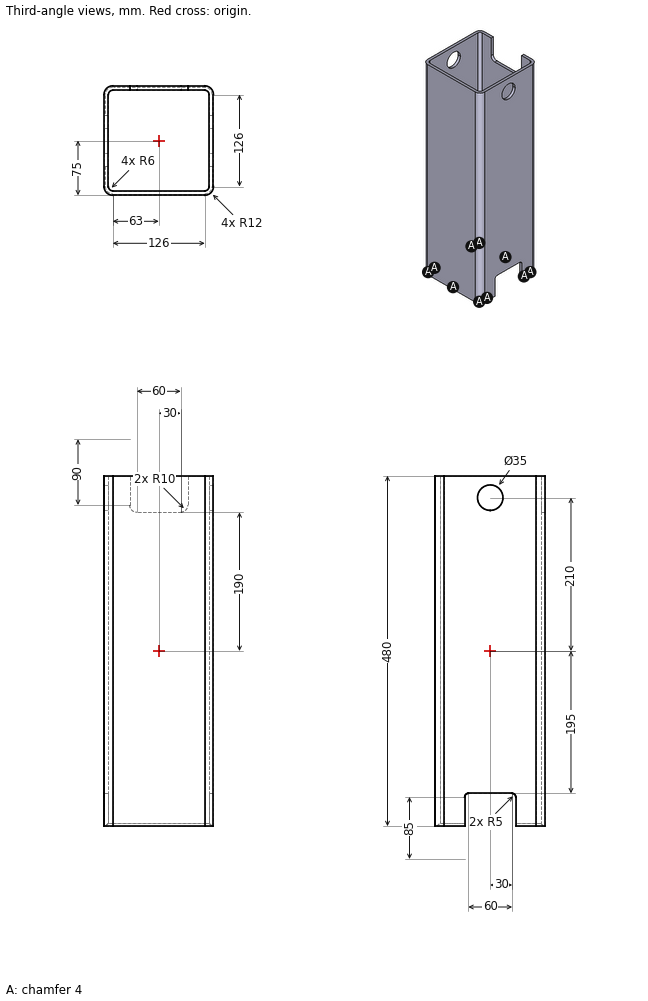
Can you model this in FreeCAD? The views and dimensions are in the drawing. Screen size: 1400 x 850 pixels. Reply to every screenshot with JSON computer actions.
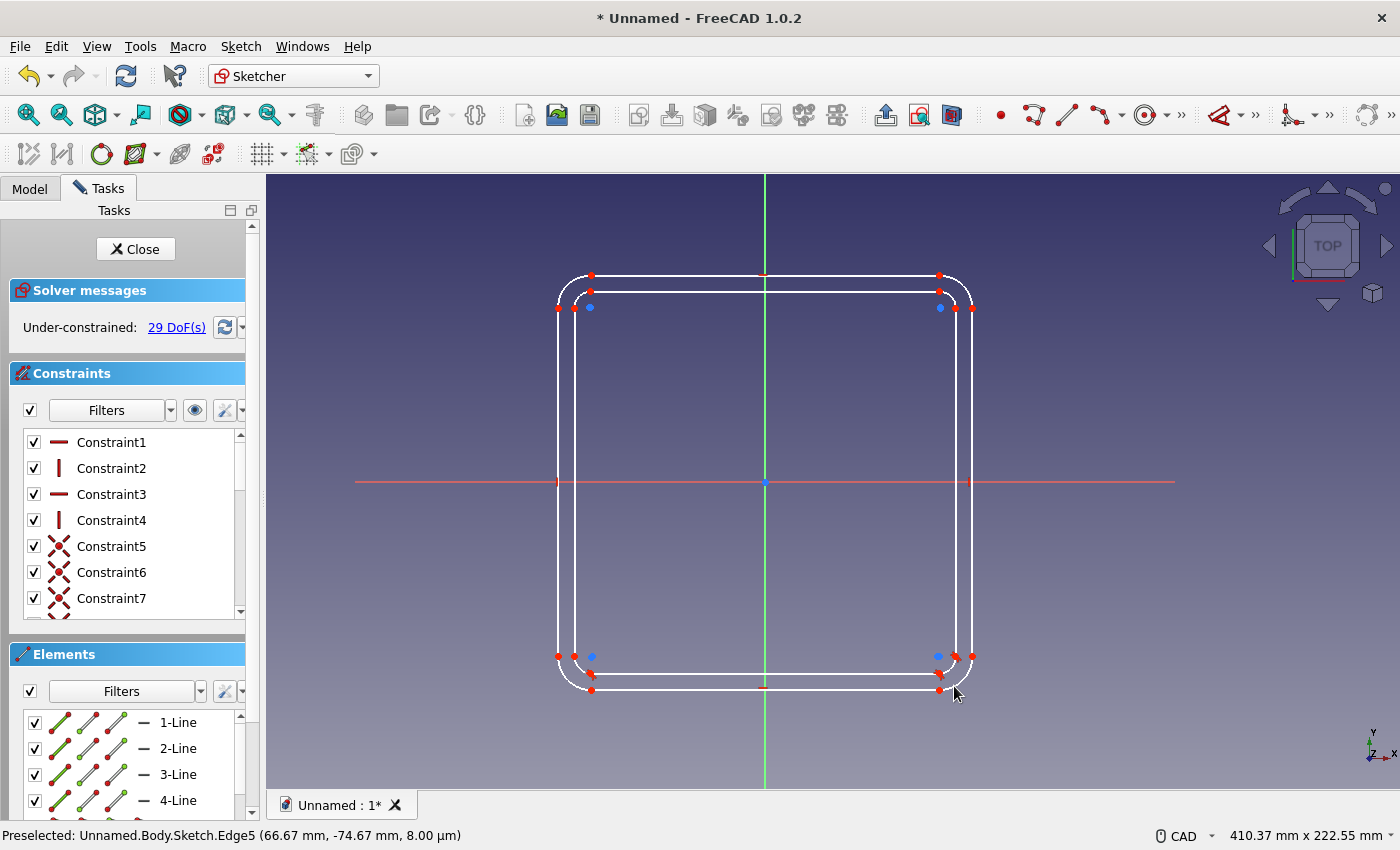
{"action": "left_click", "coordinate": [972, 553]}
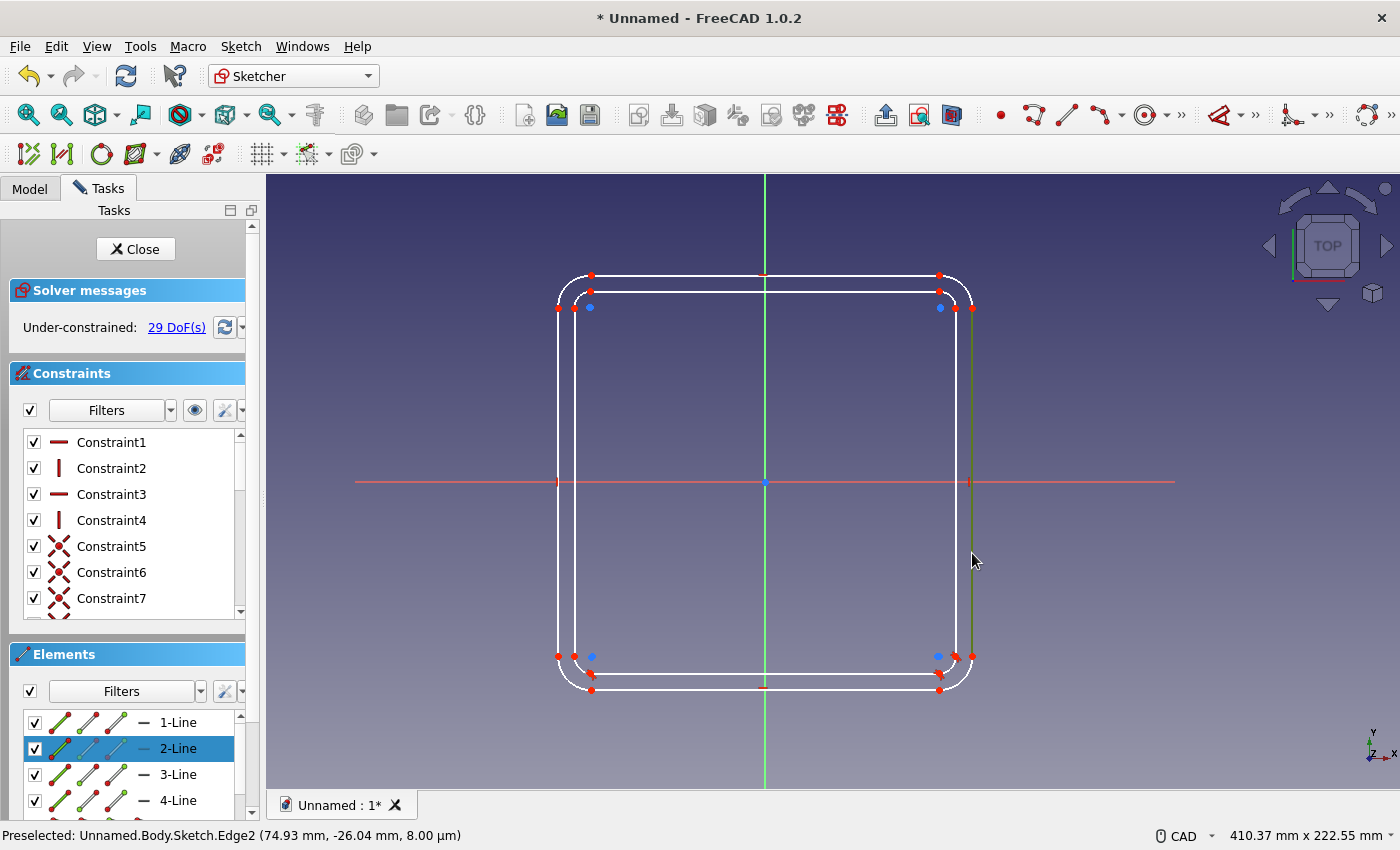
{"action": "left_click", "coordinate": [969, 294]}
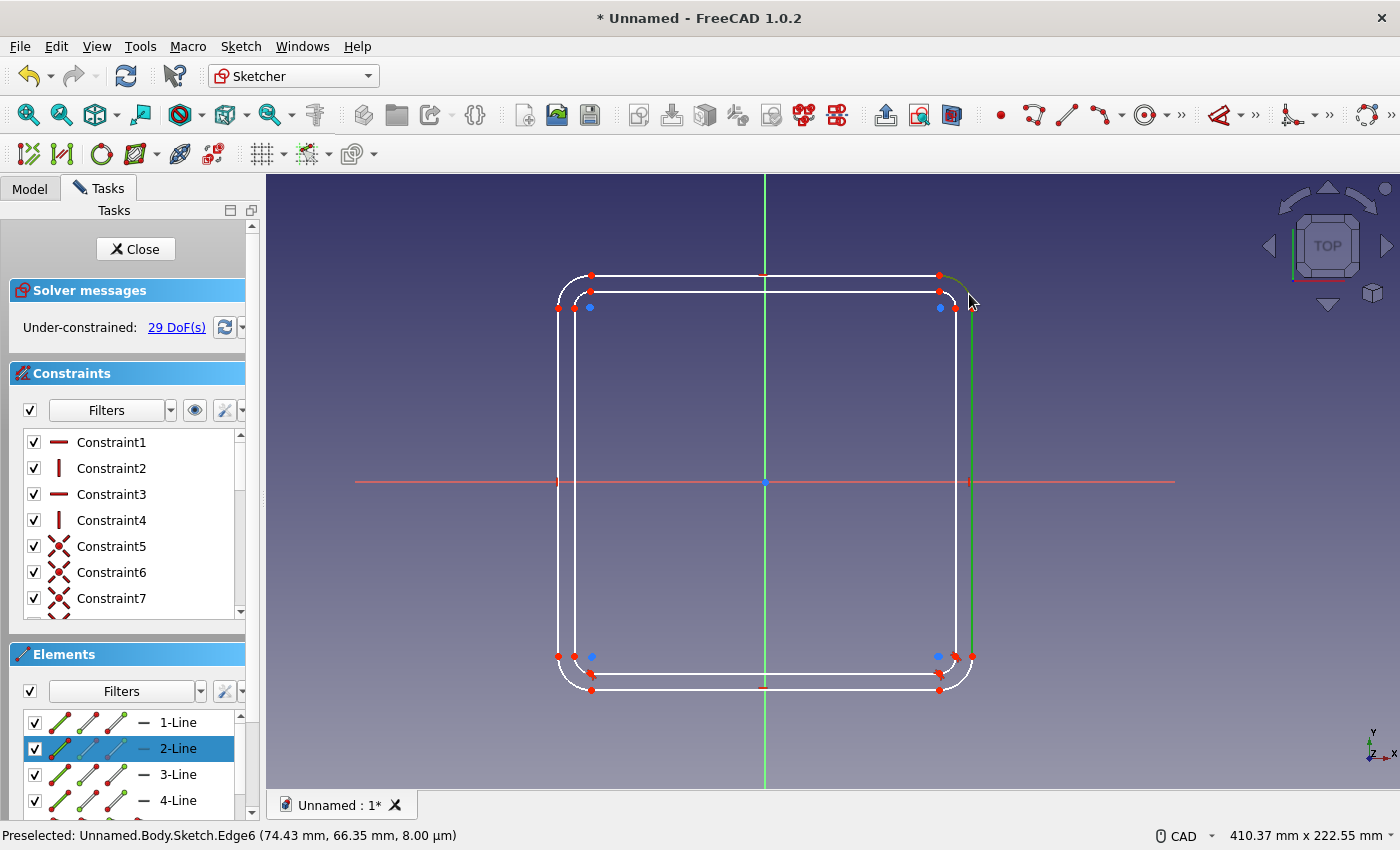
{"action": "key", "text": "t"}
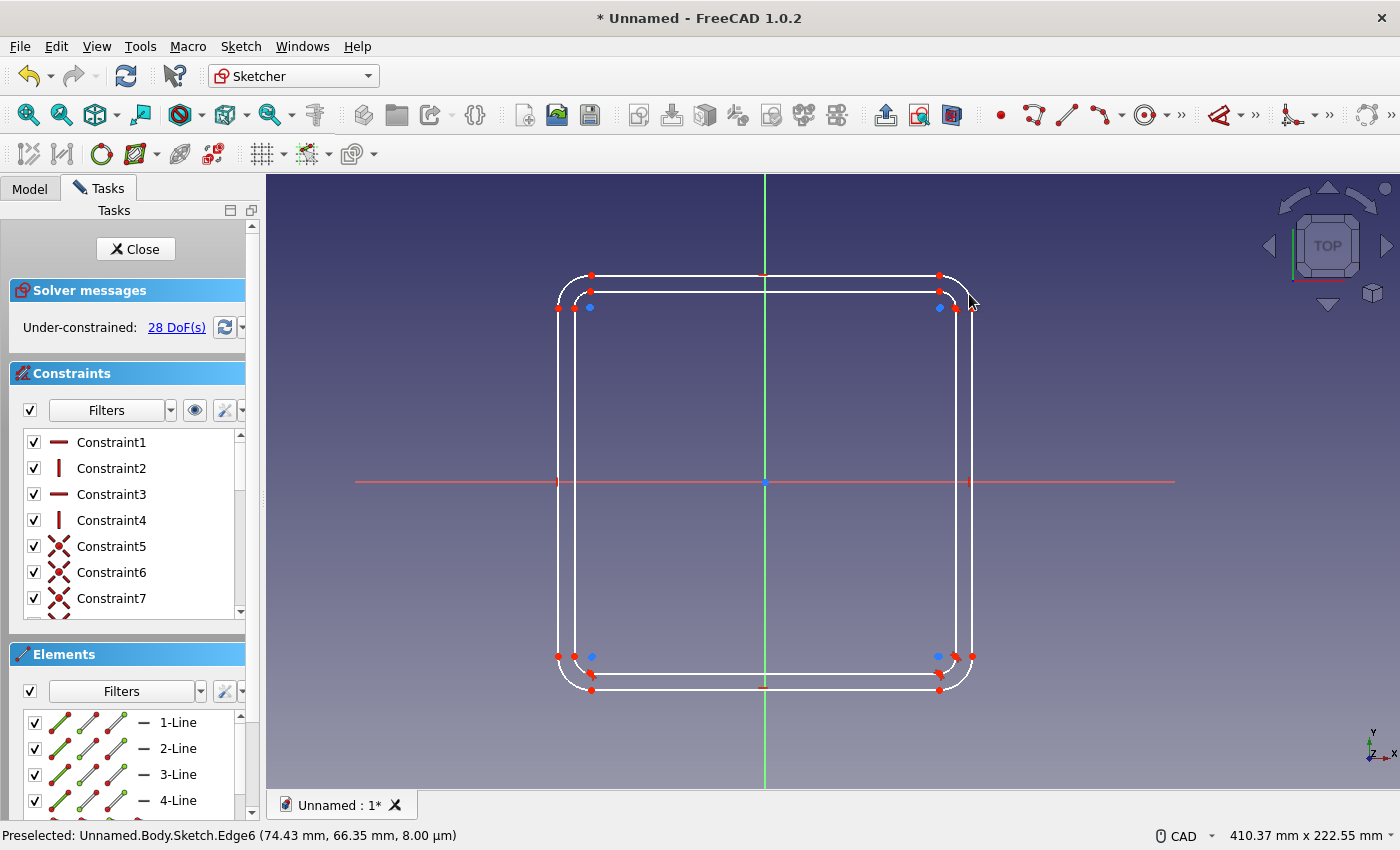
{"action": "left_click", "coordinate": [835, 276]}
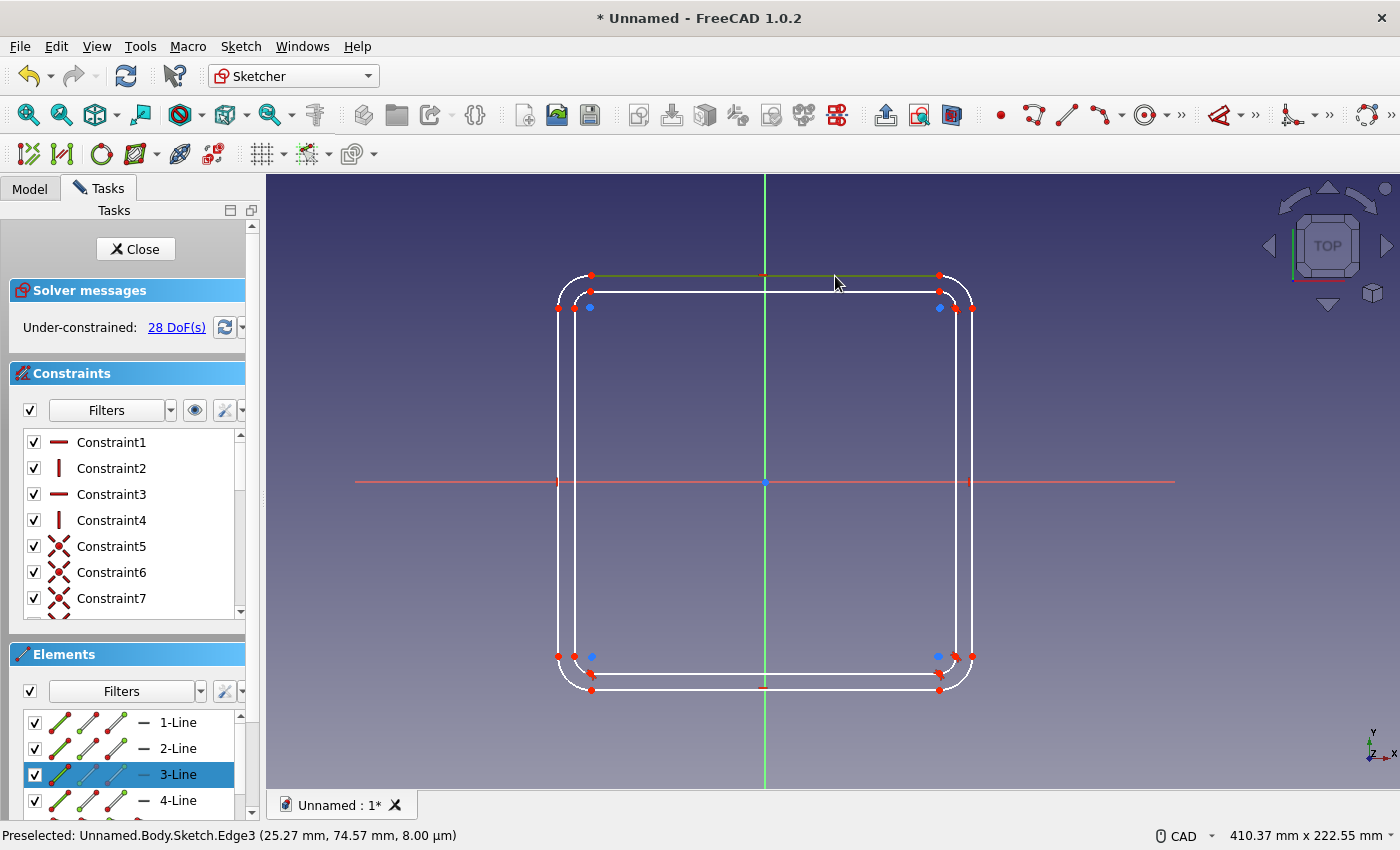
{"action": "left_click", "coordinate": [969, 294]}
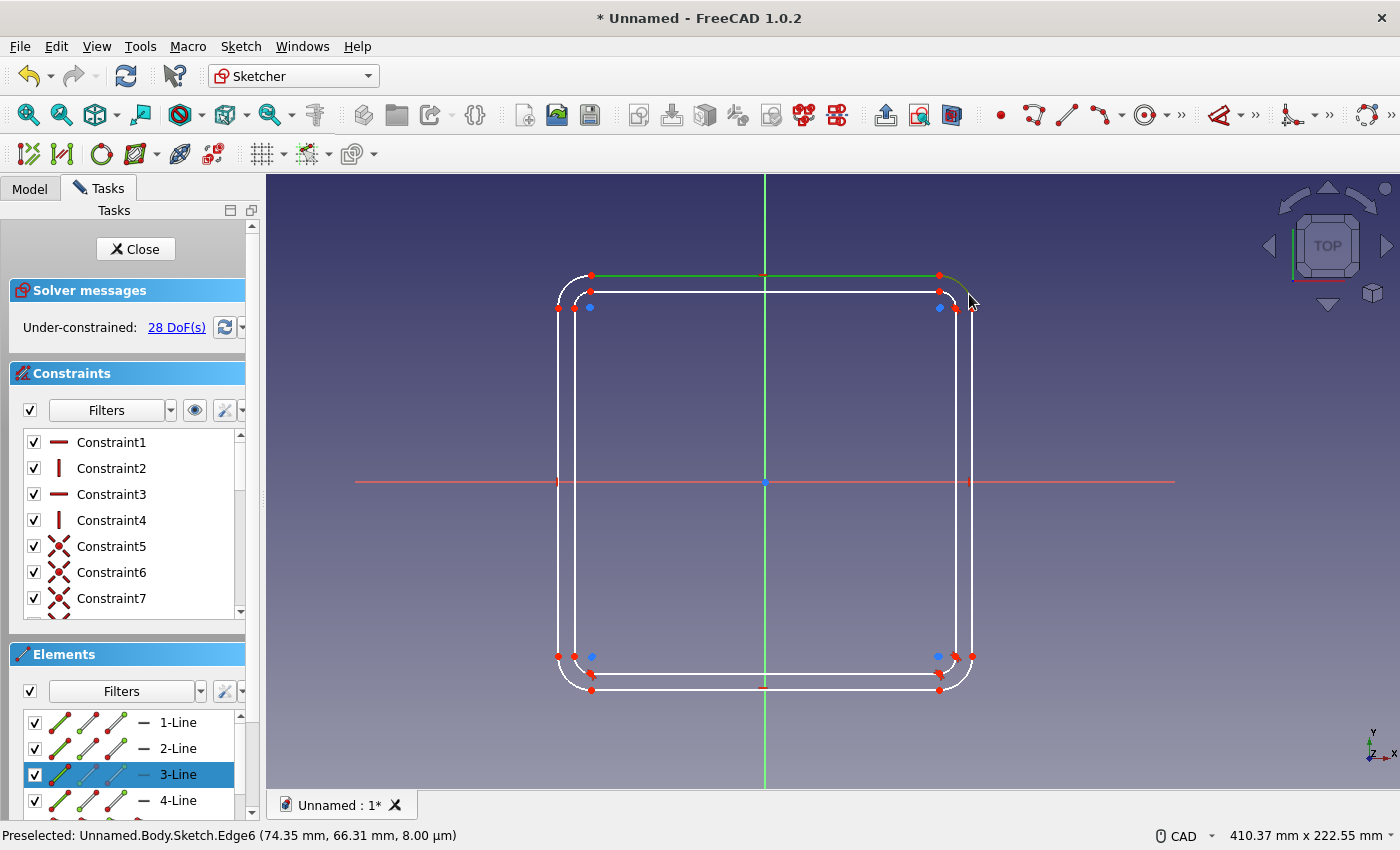
{"action": "key", "text": "t"}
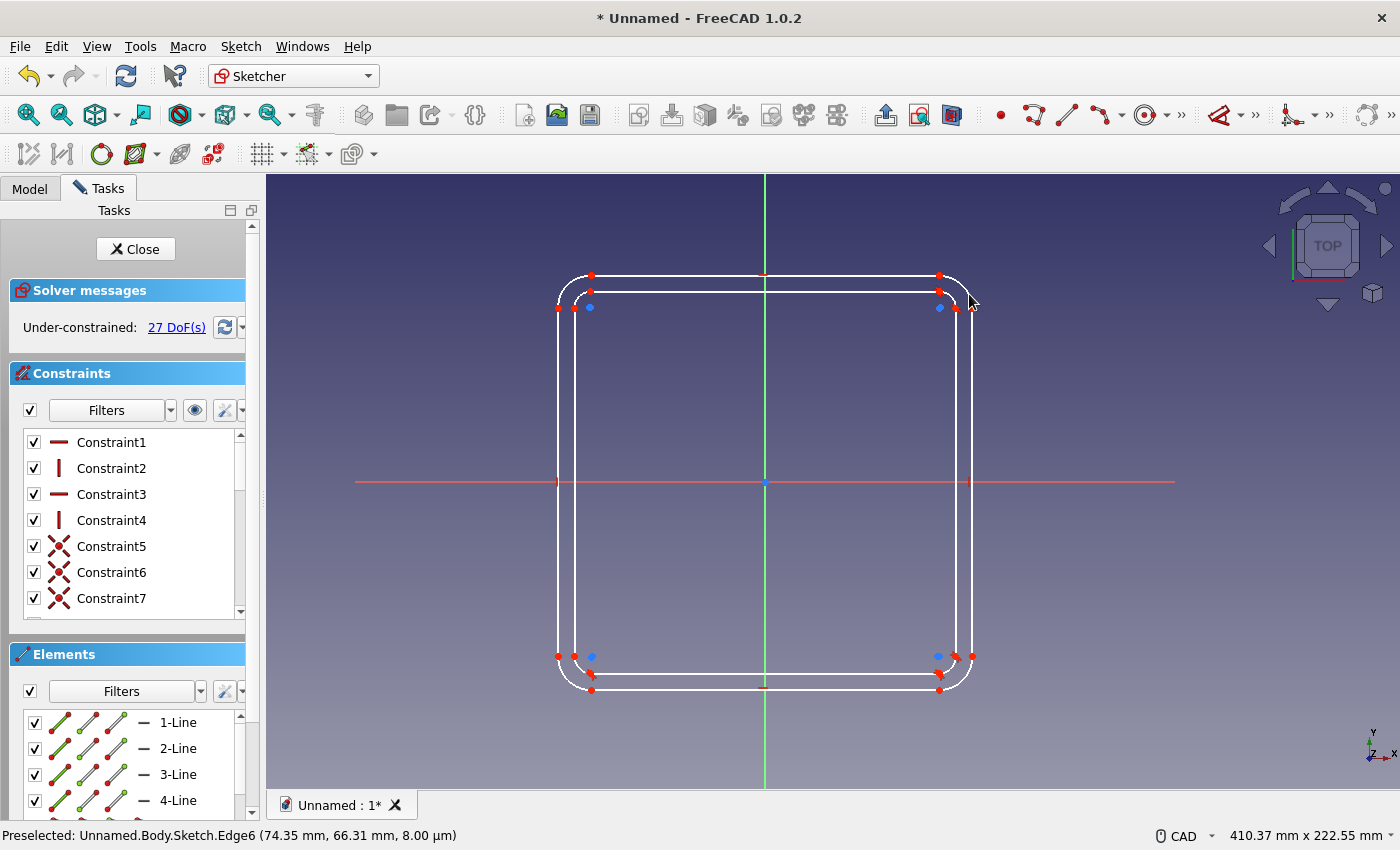
{"action": "left_click", "coordinate": [835, 276]}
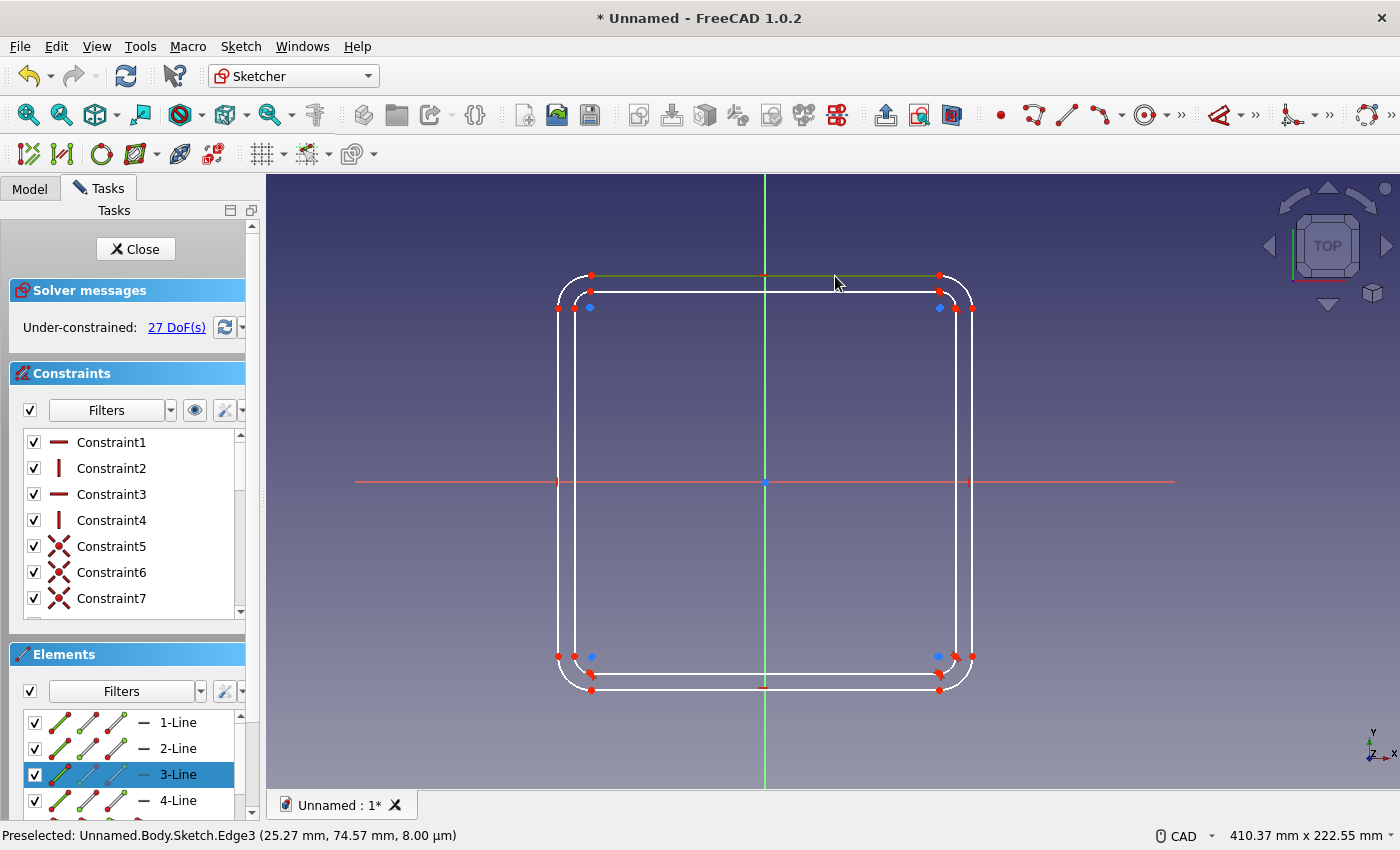
{"action": "left_click", "coordinate": [576, 279]}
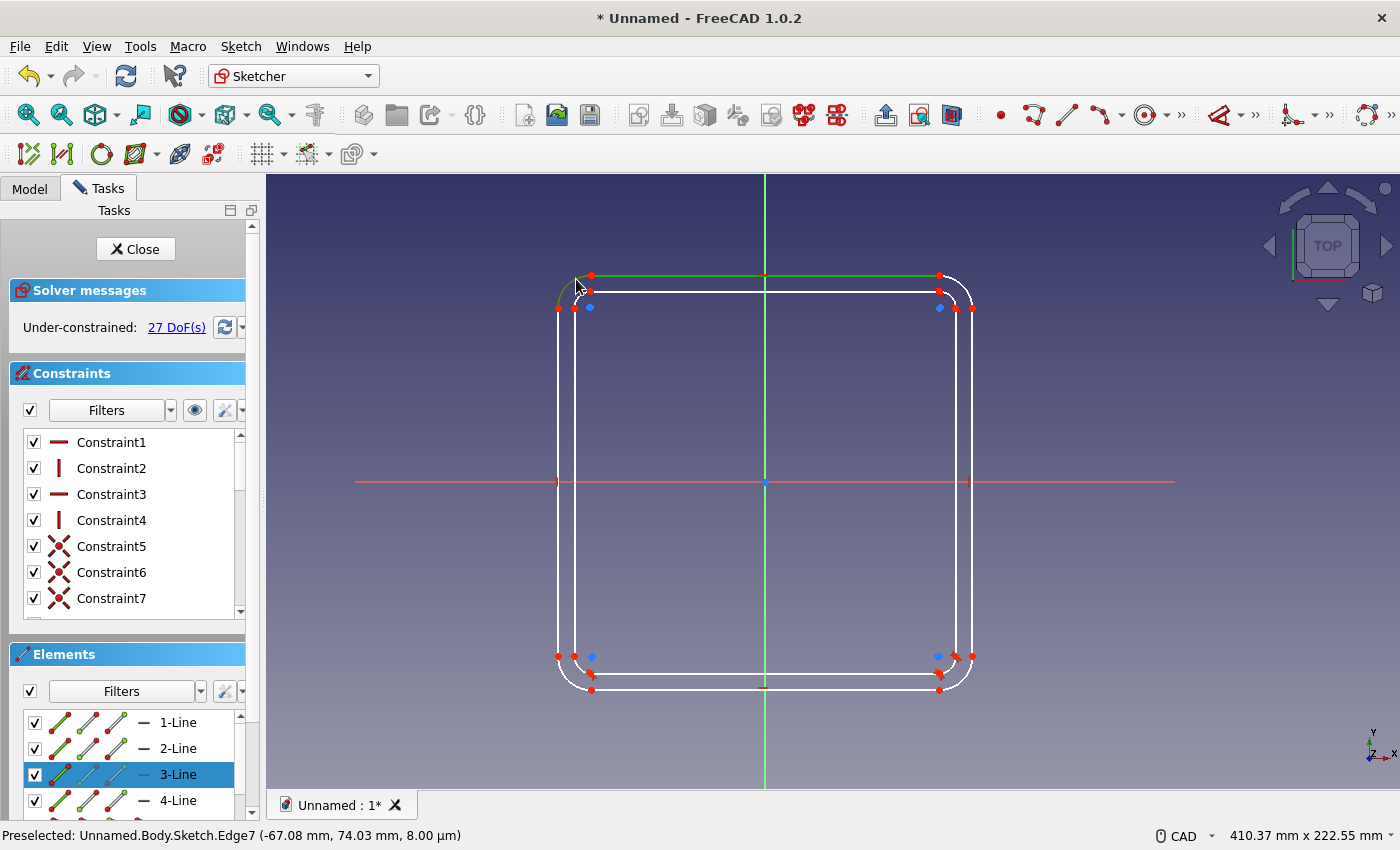
{"action": "key", "text": "t"}